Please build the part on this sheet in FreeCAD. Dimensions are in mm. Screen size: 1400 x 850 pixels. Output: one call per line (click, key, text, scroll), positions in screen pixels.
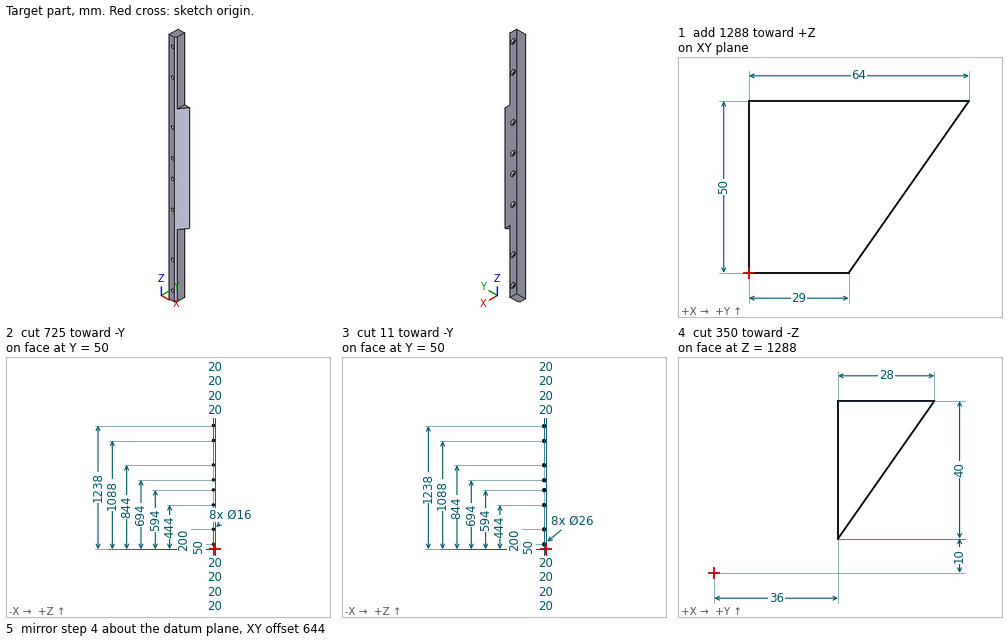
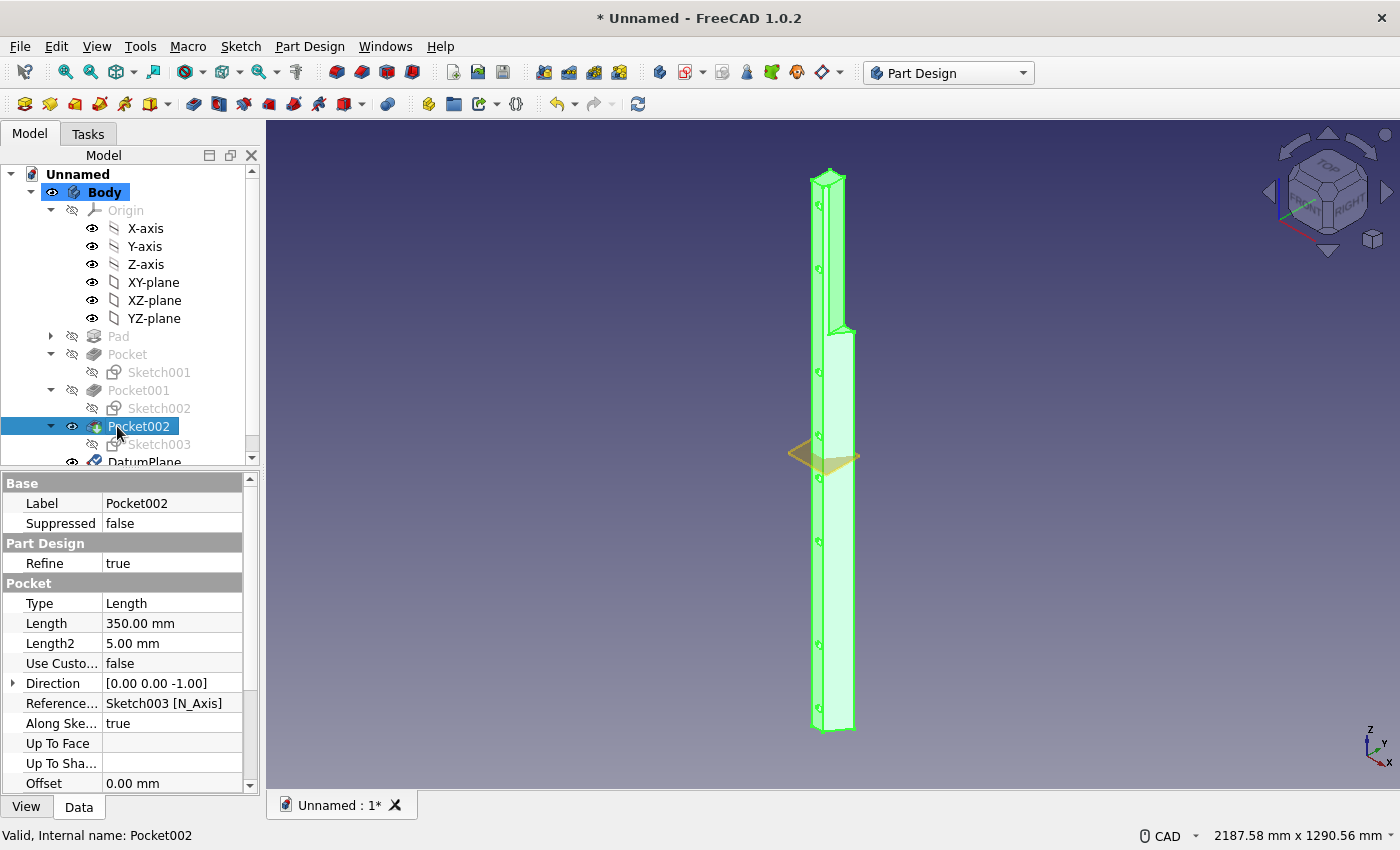
click(544, 72)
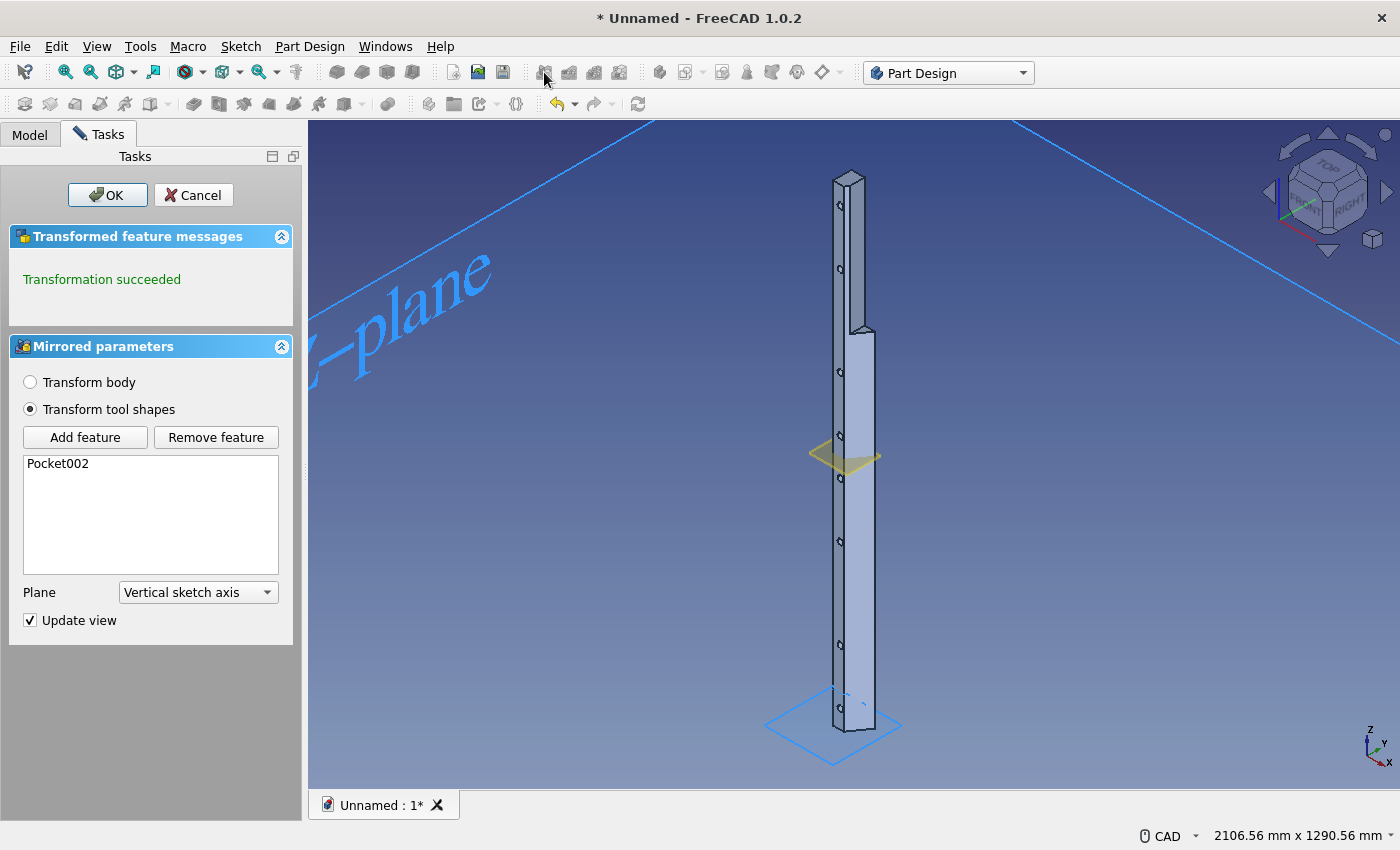
click(199, 592)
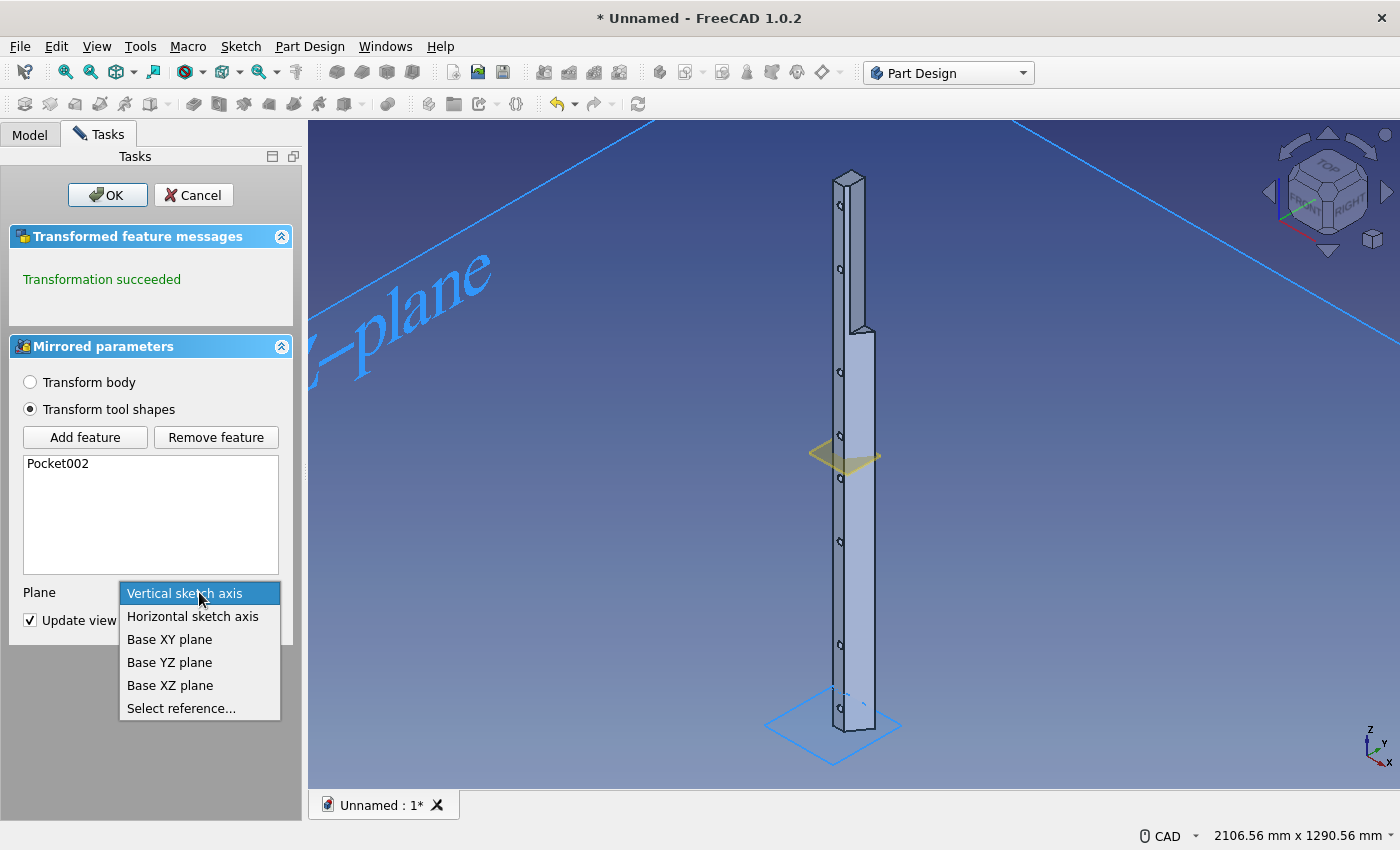
click(198, 708)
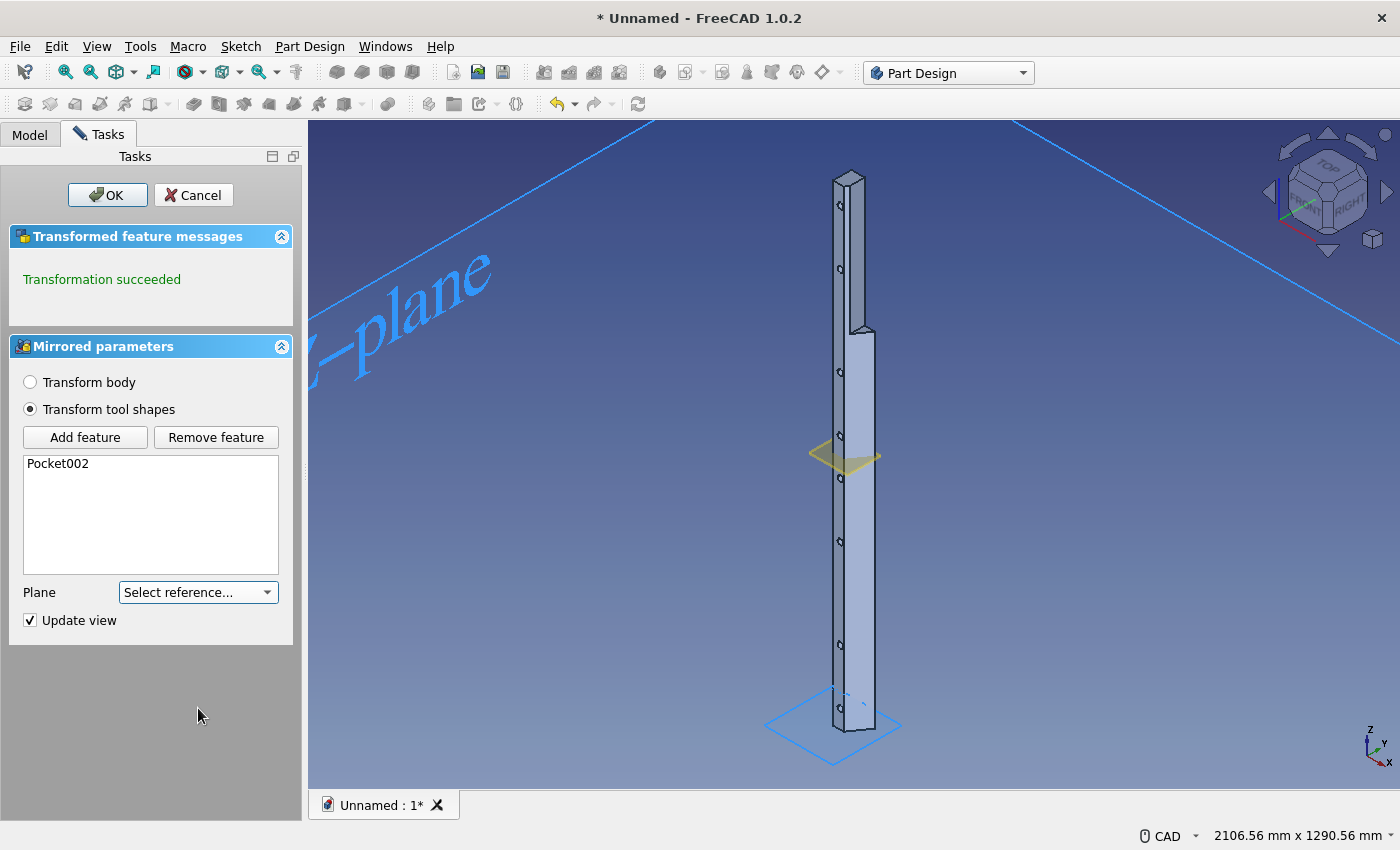
click(30, 134)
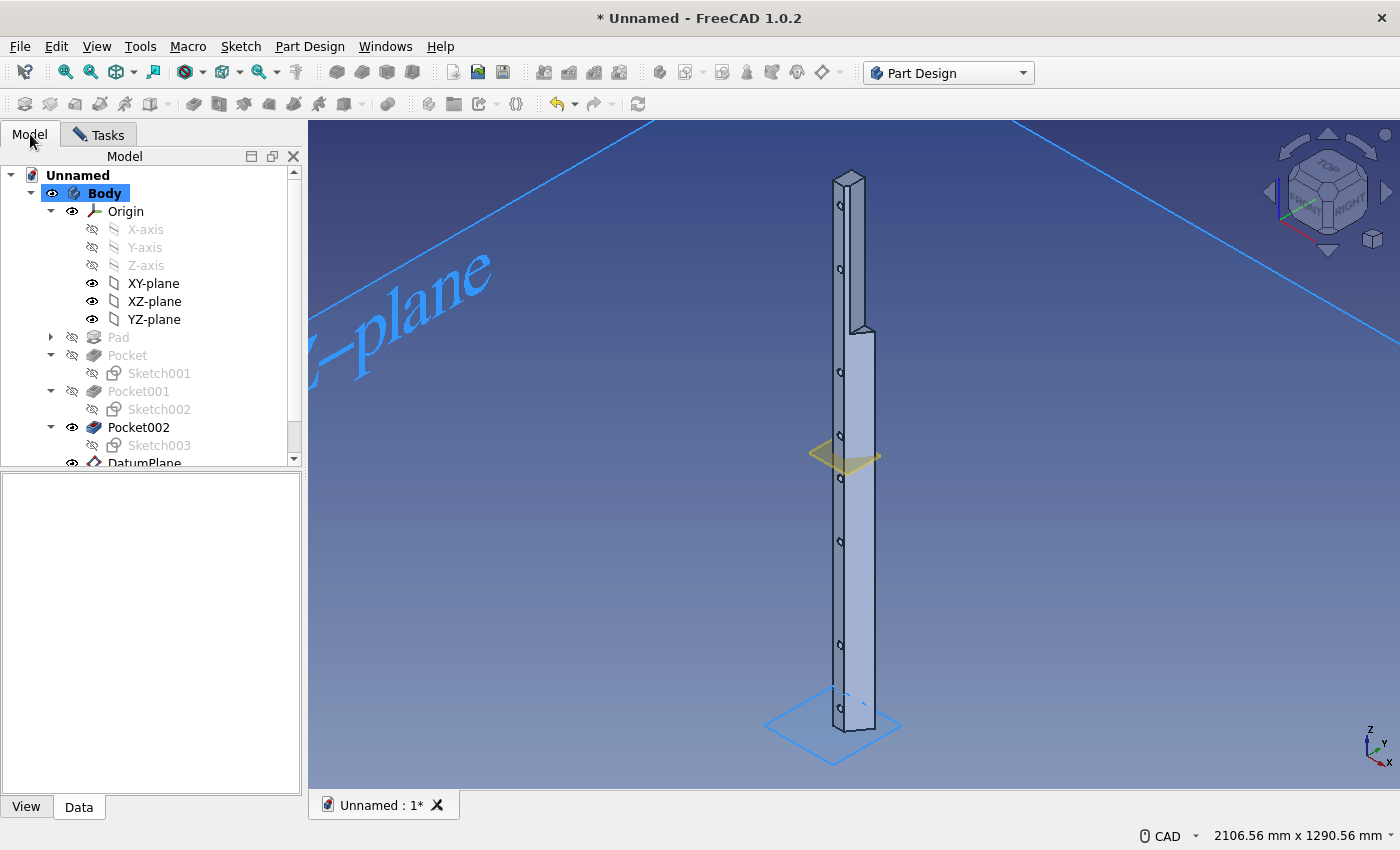
click(117, 463)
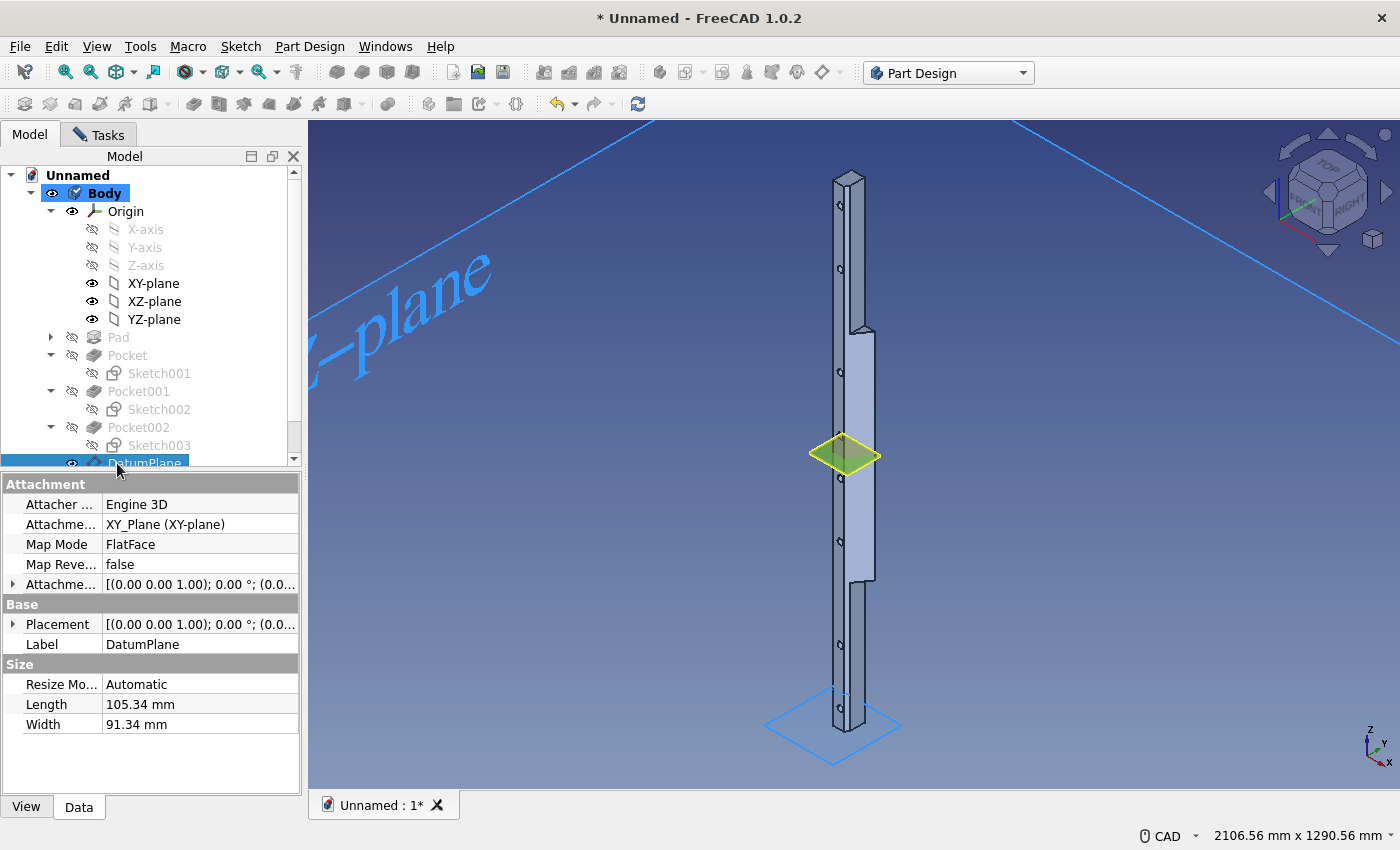
click(98, 134)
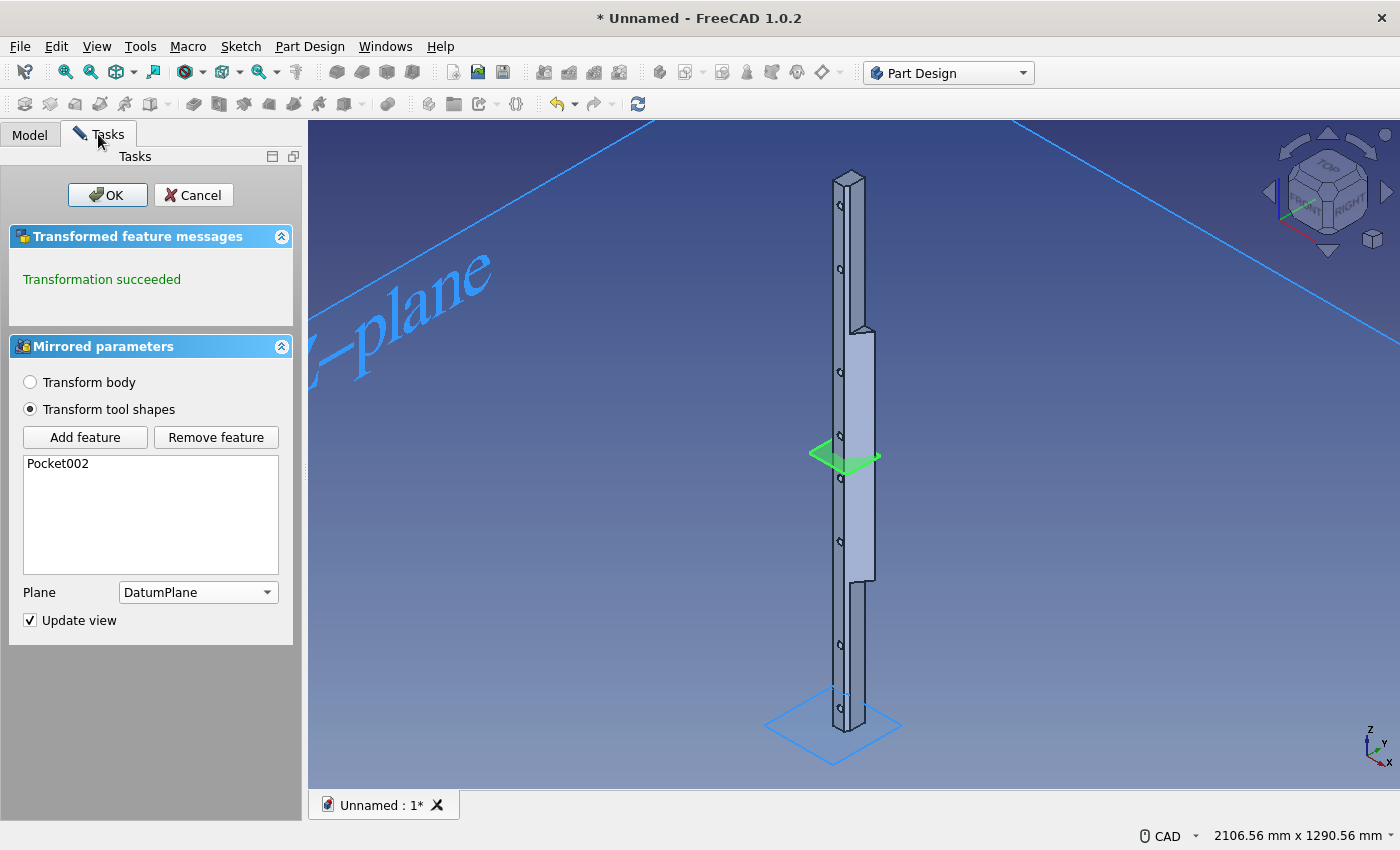
click(108, 195)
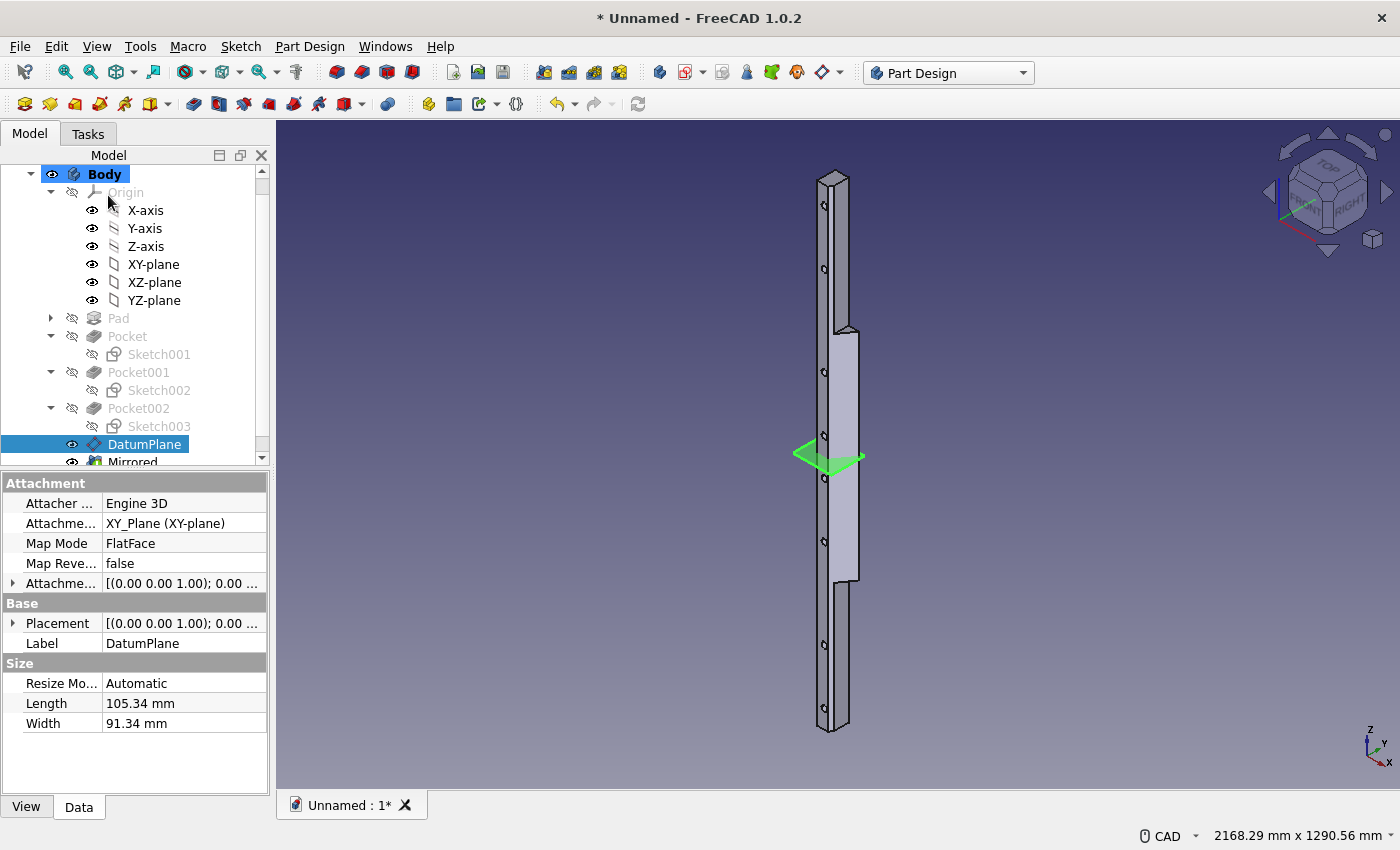
click(117, 444)
key(space)